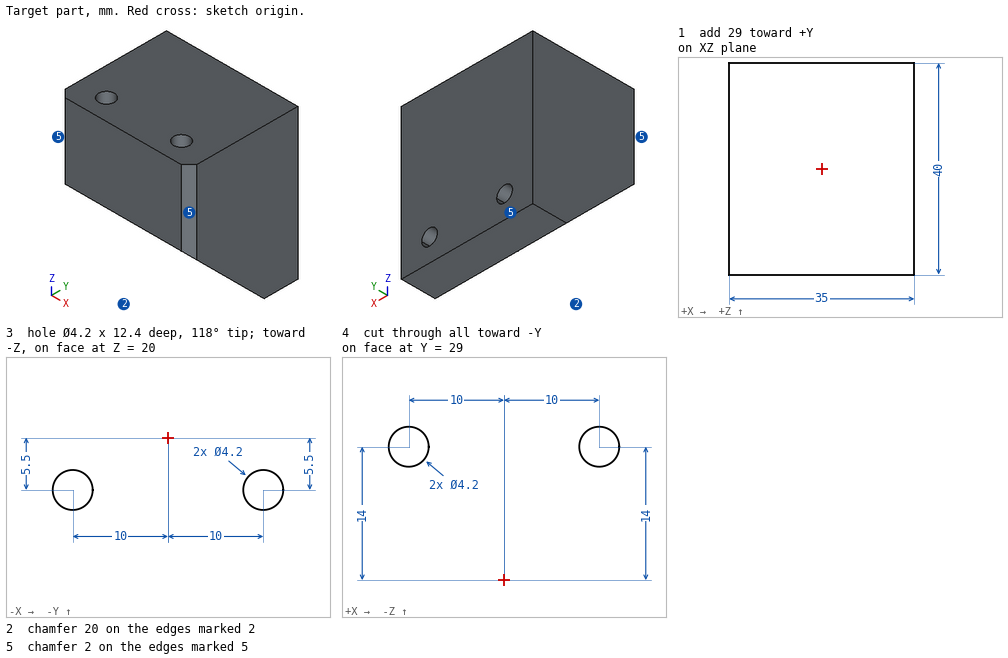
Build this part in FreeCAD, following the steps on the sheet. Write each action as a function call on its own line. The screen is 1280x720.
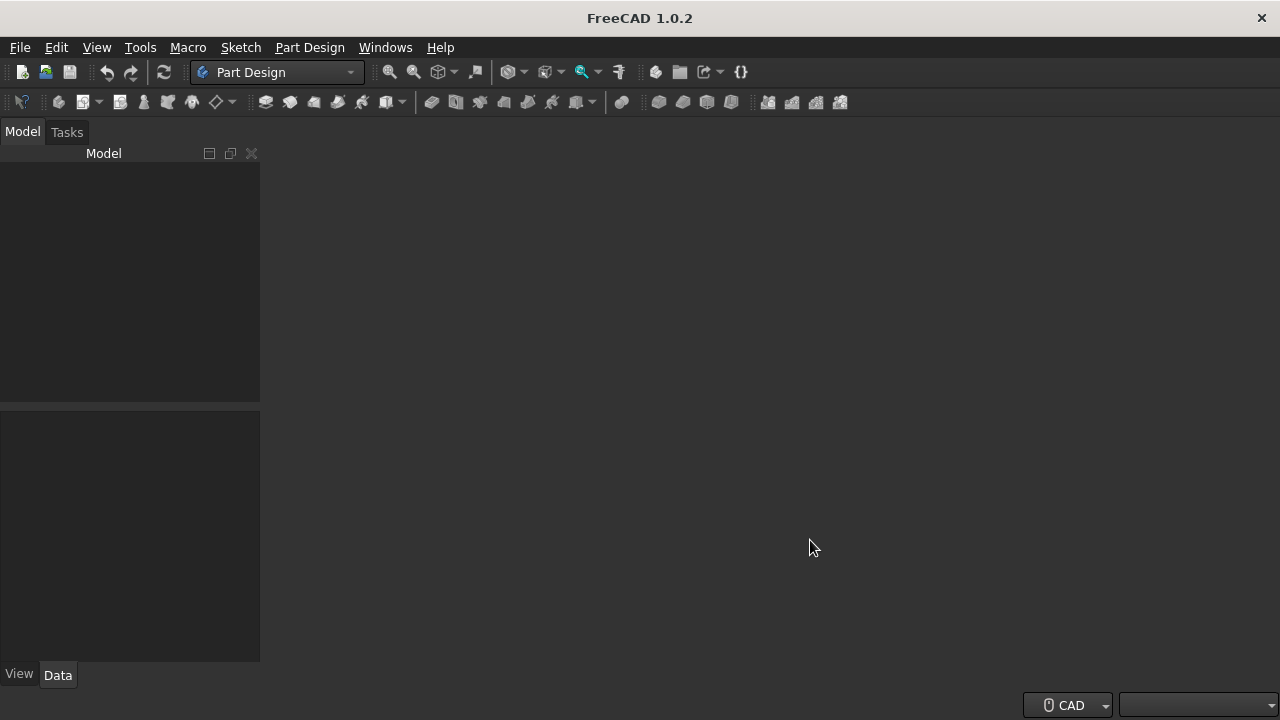
key(ctrl+n)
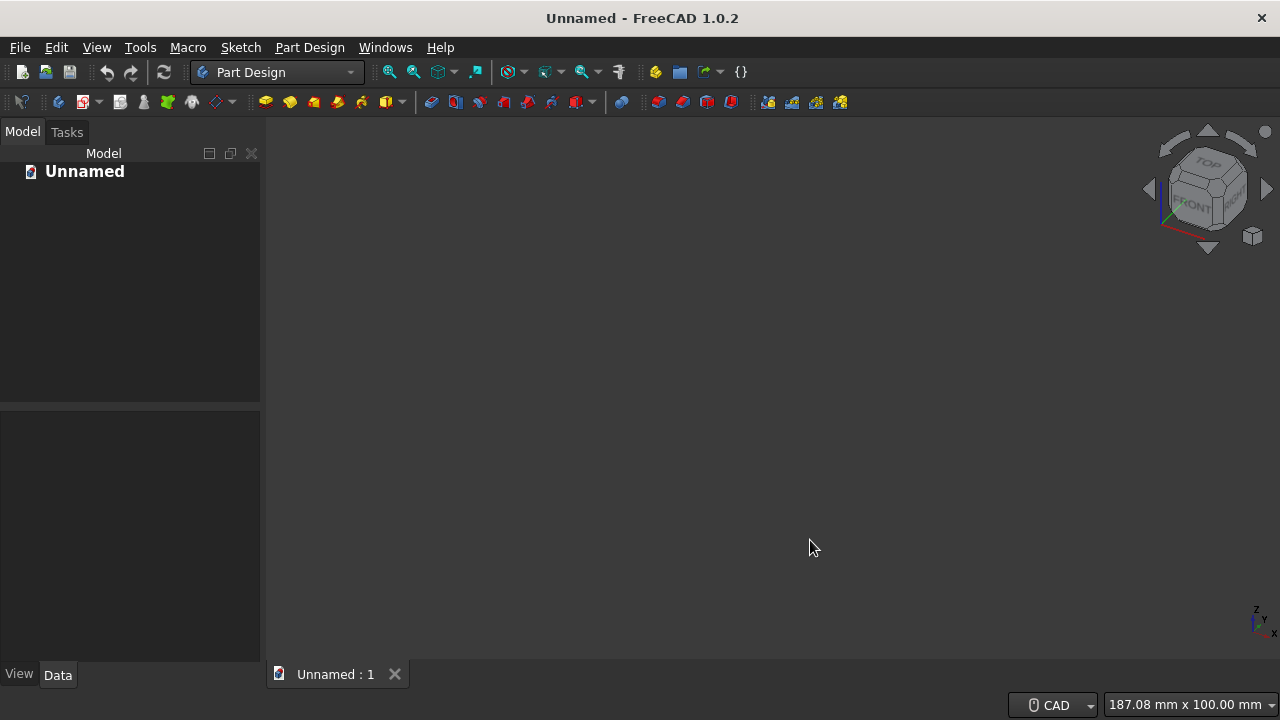
click(84, 102)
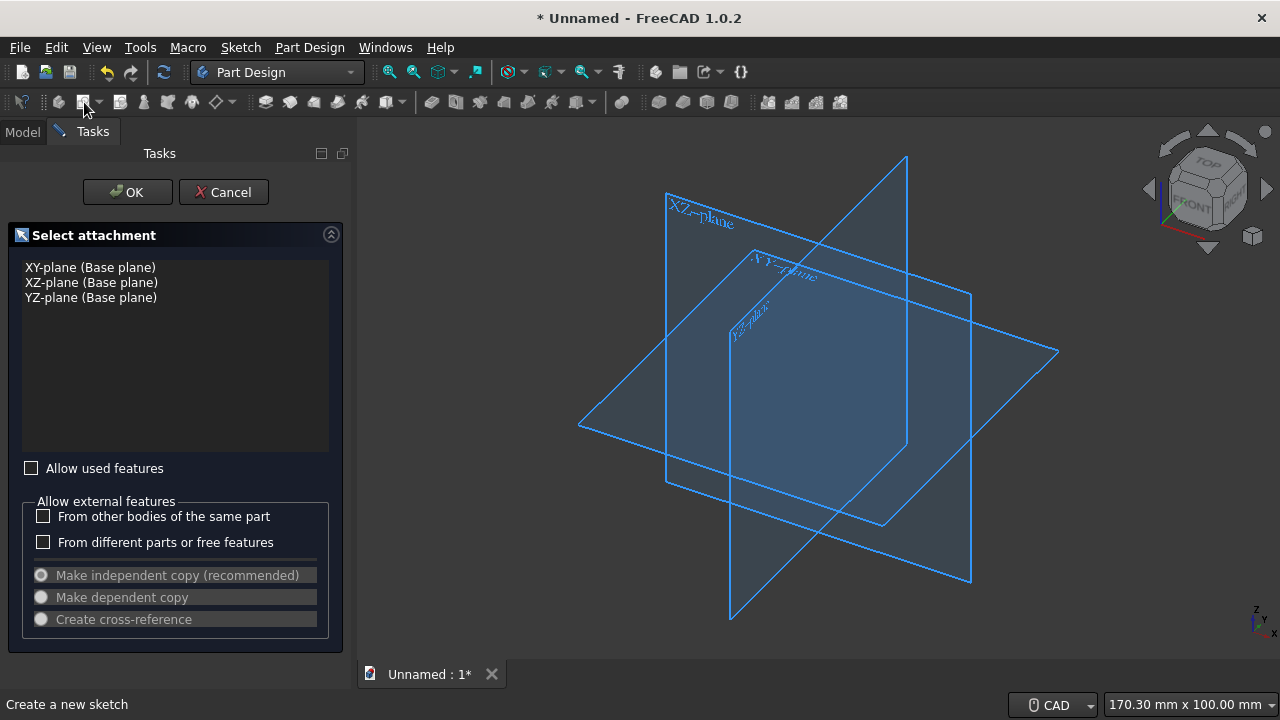
click(82, 282)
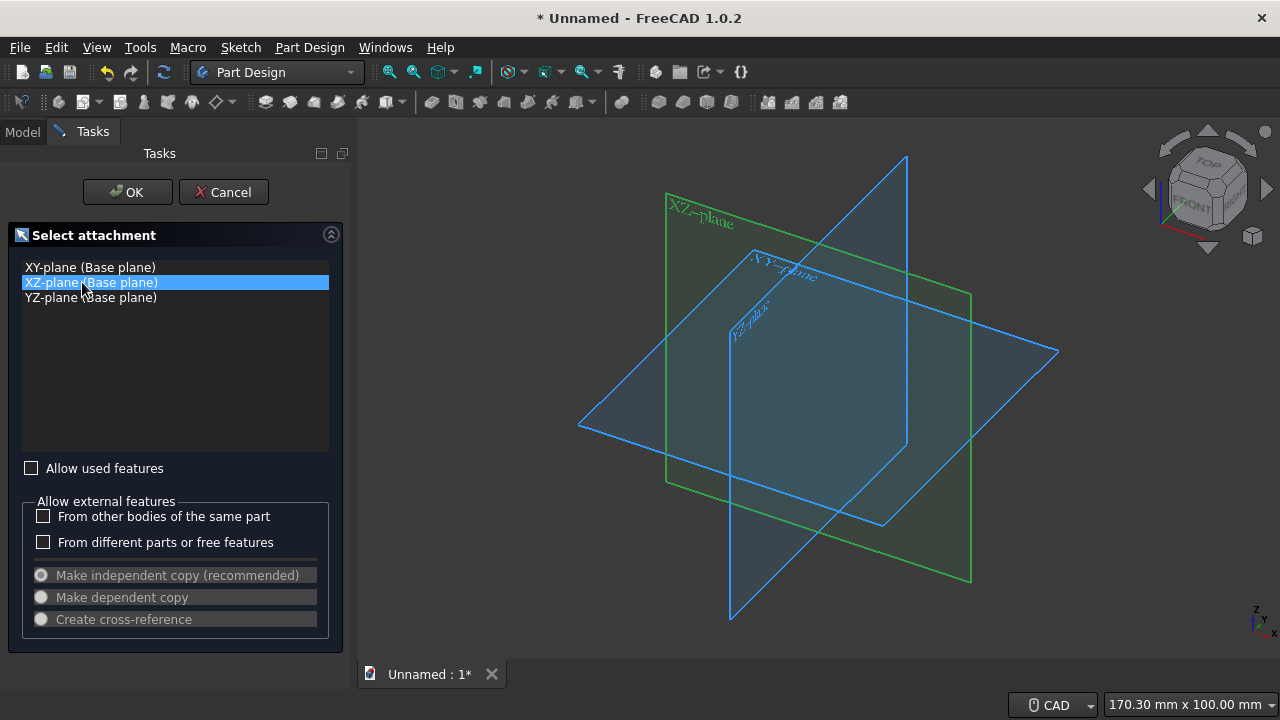
click(128, 192)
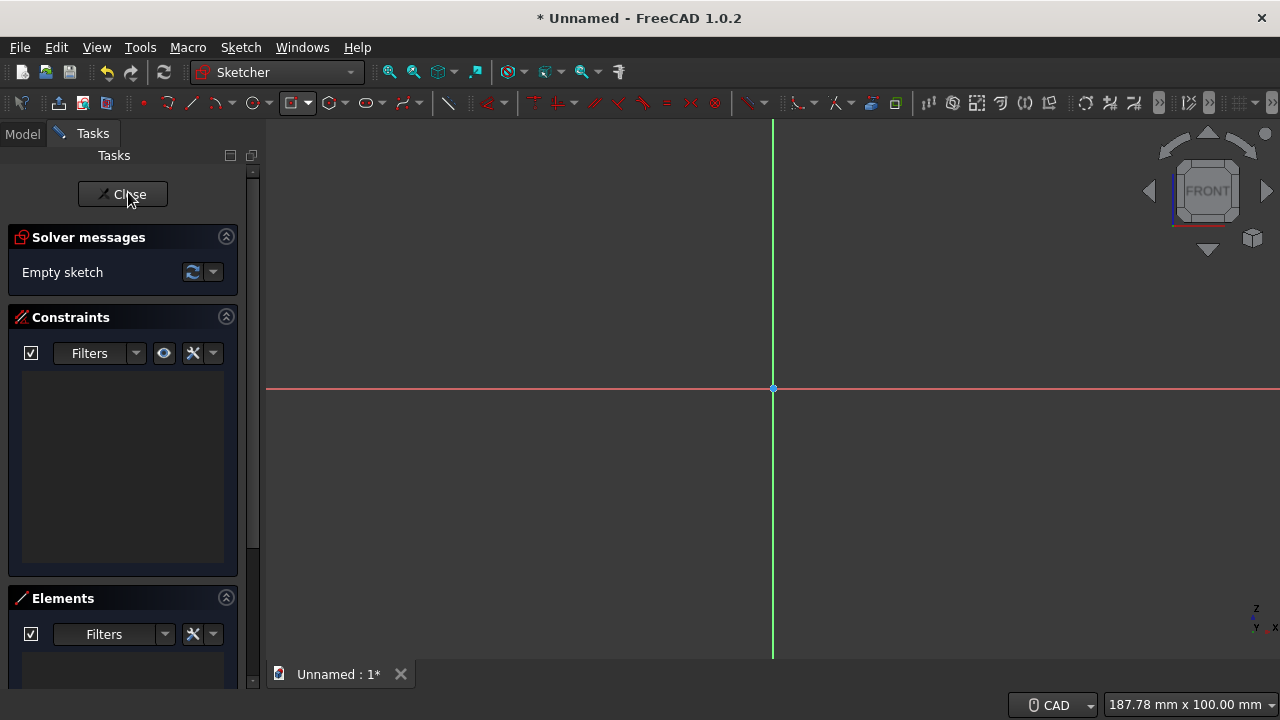
scroll(912, 389, up, 2)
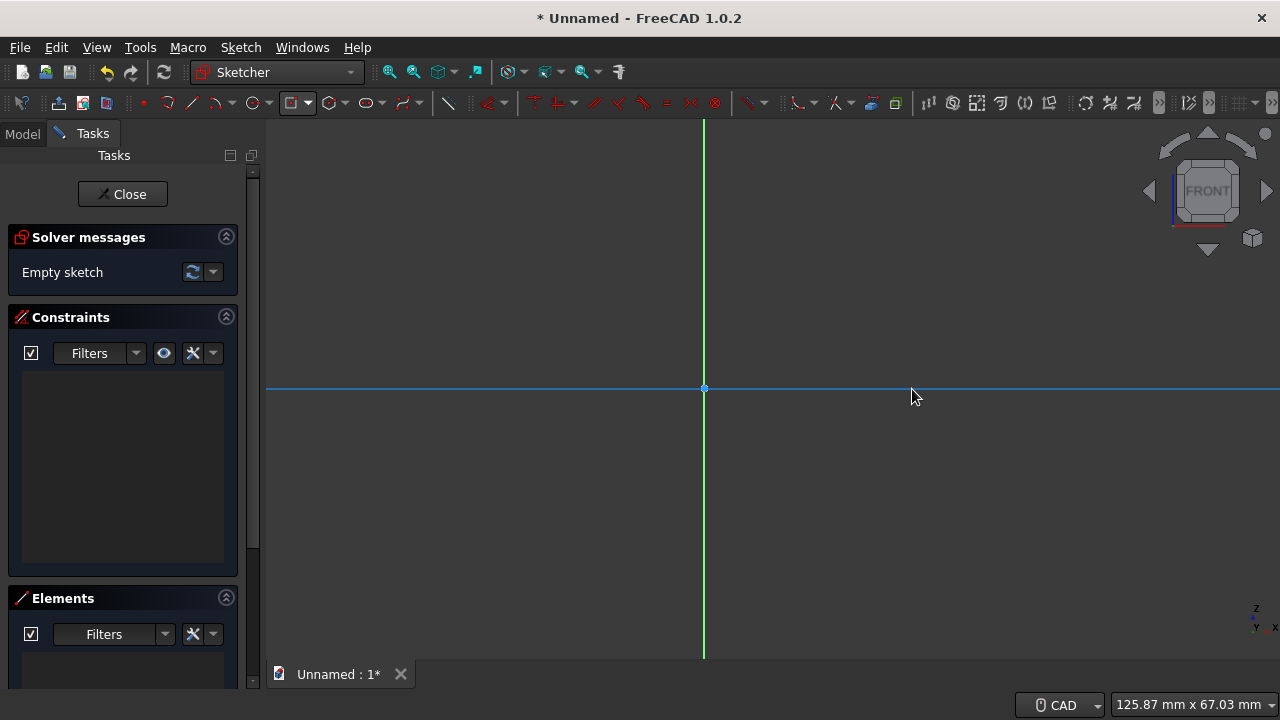
key(g)
key(v)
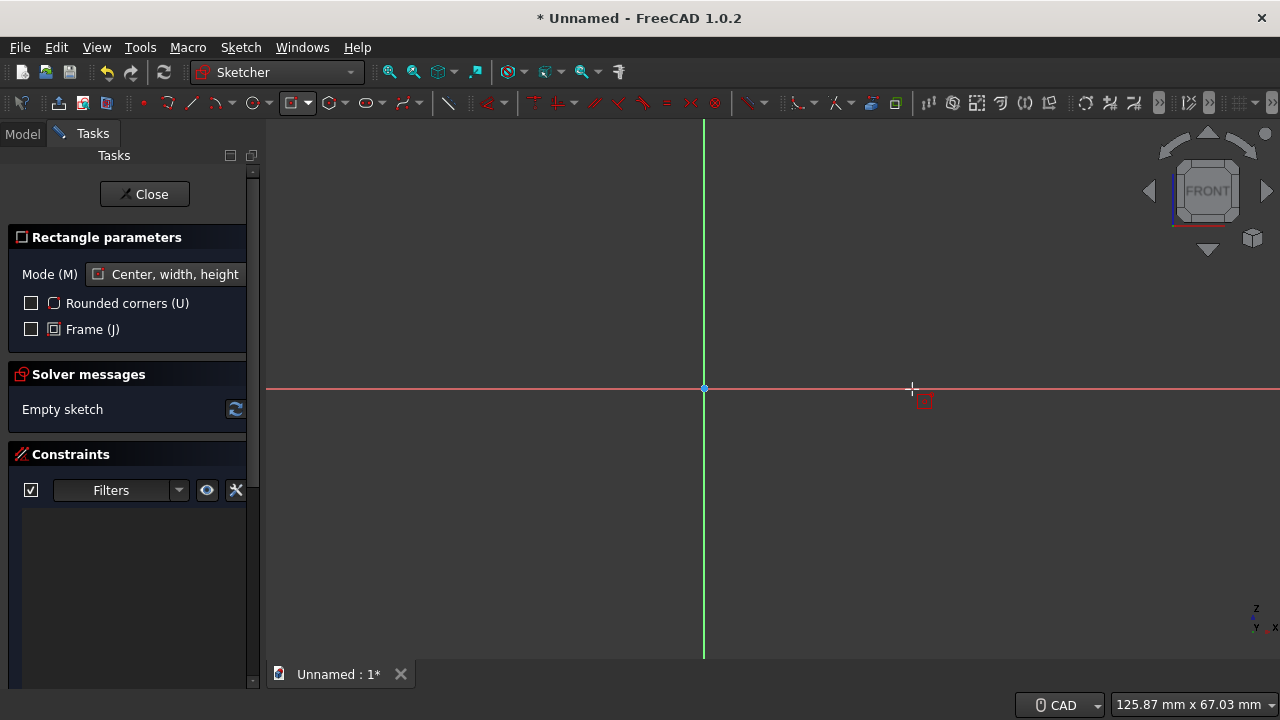
click(704, 389)
move(845, 228)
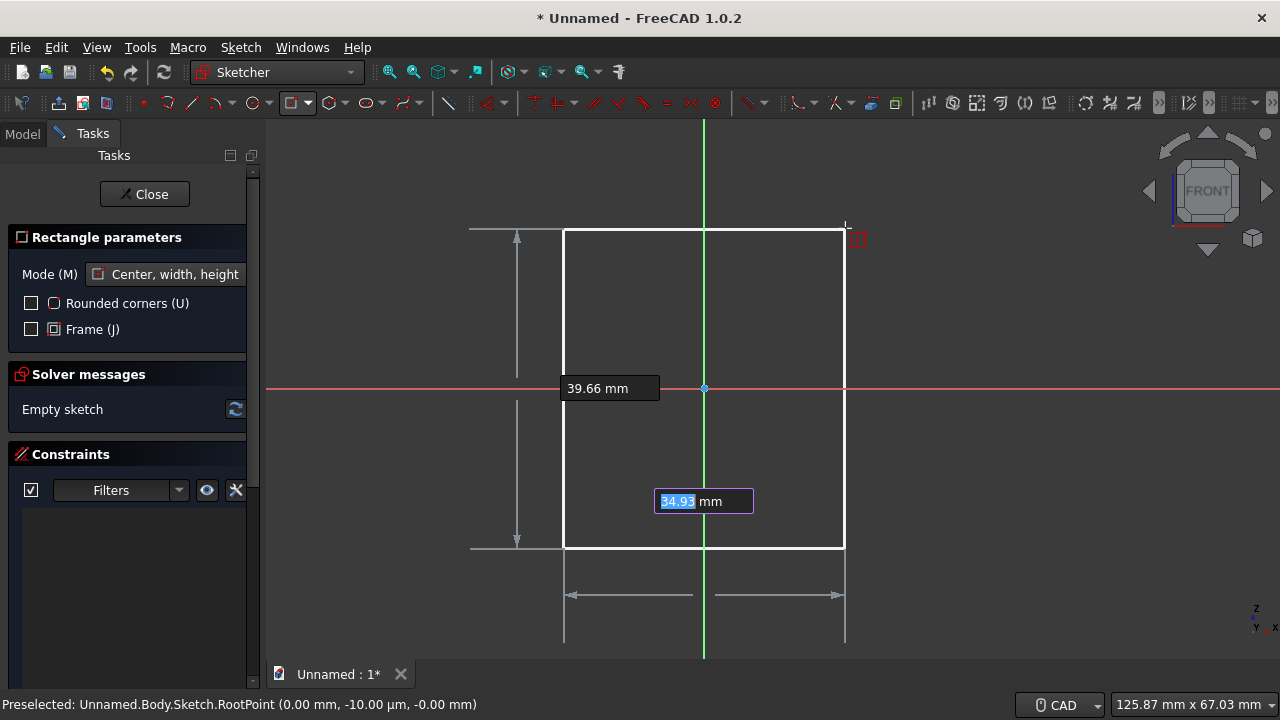
text(35)
key(Tab)
text(40)
key(Return)
key(Escape)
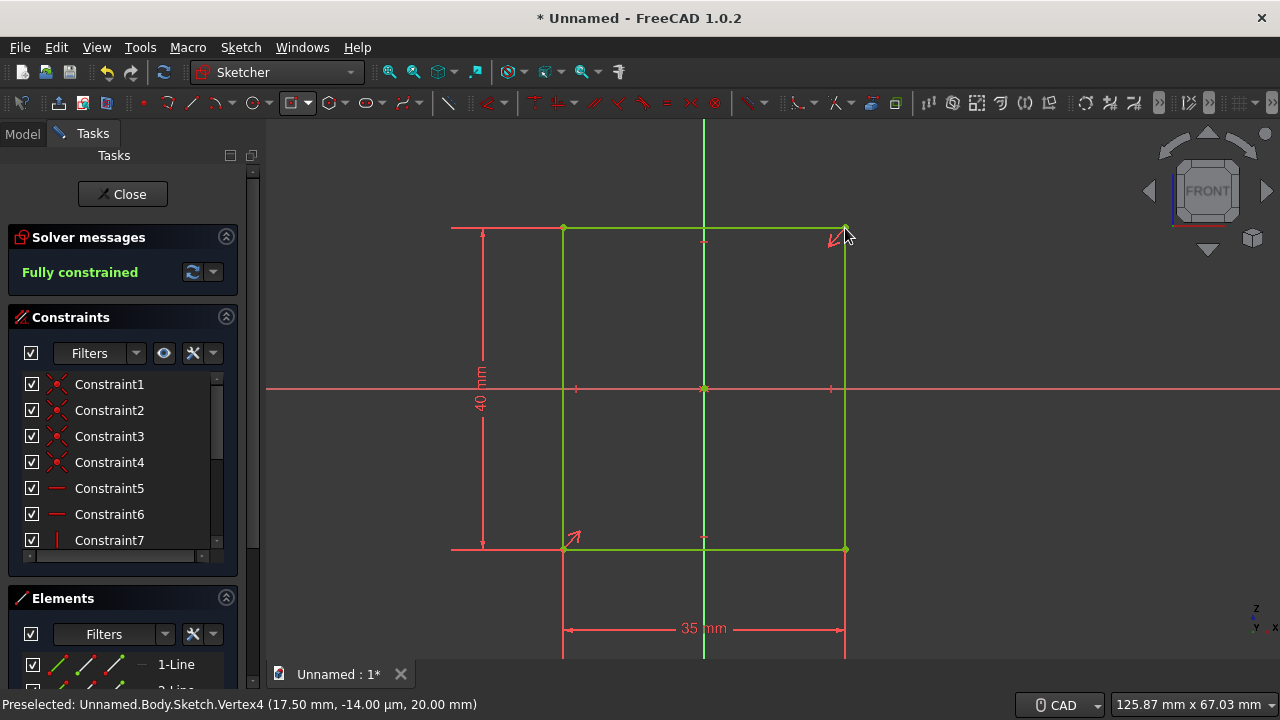
click(123, 194)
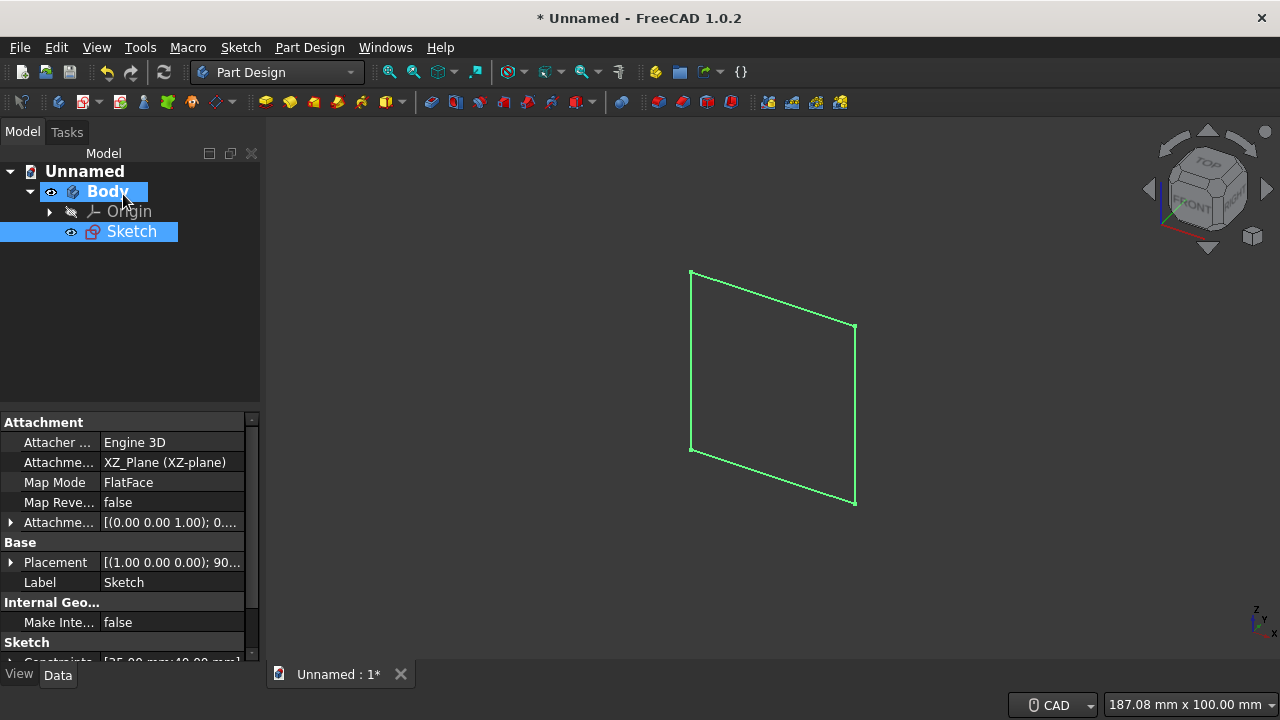
click(266, 102)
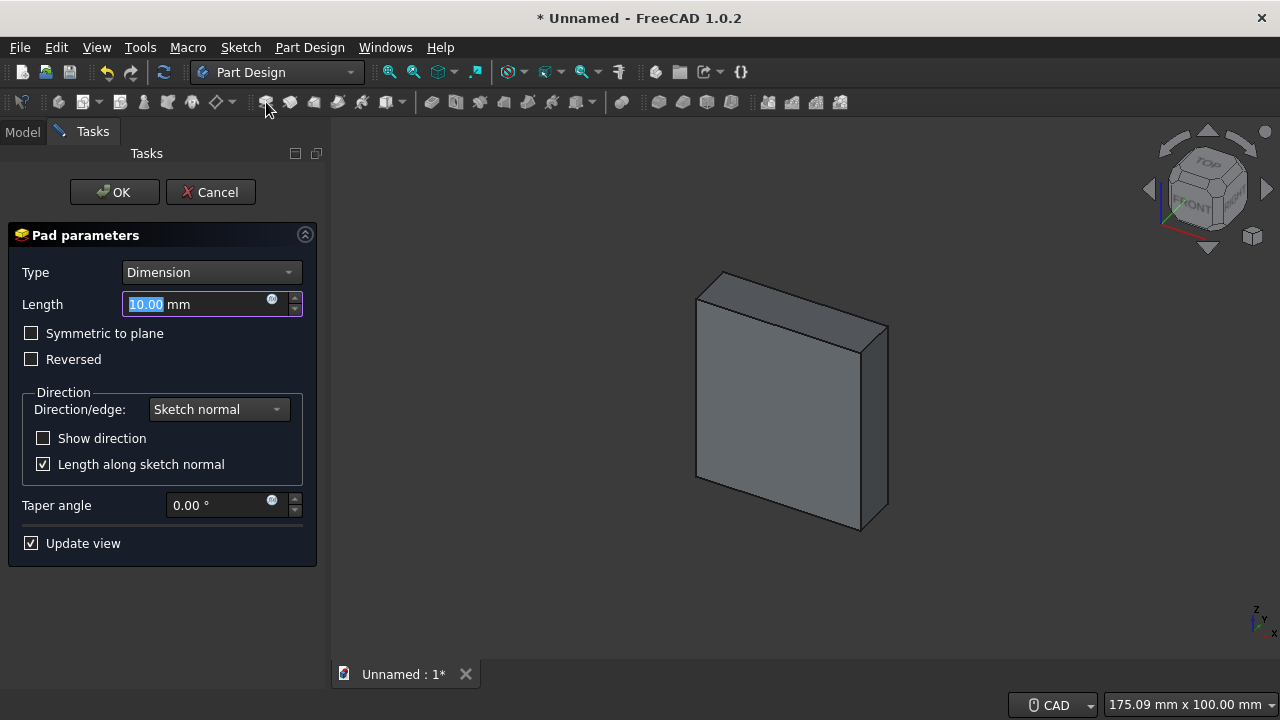
text(29)
key(Tab)